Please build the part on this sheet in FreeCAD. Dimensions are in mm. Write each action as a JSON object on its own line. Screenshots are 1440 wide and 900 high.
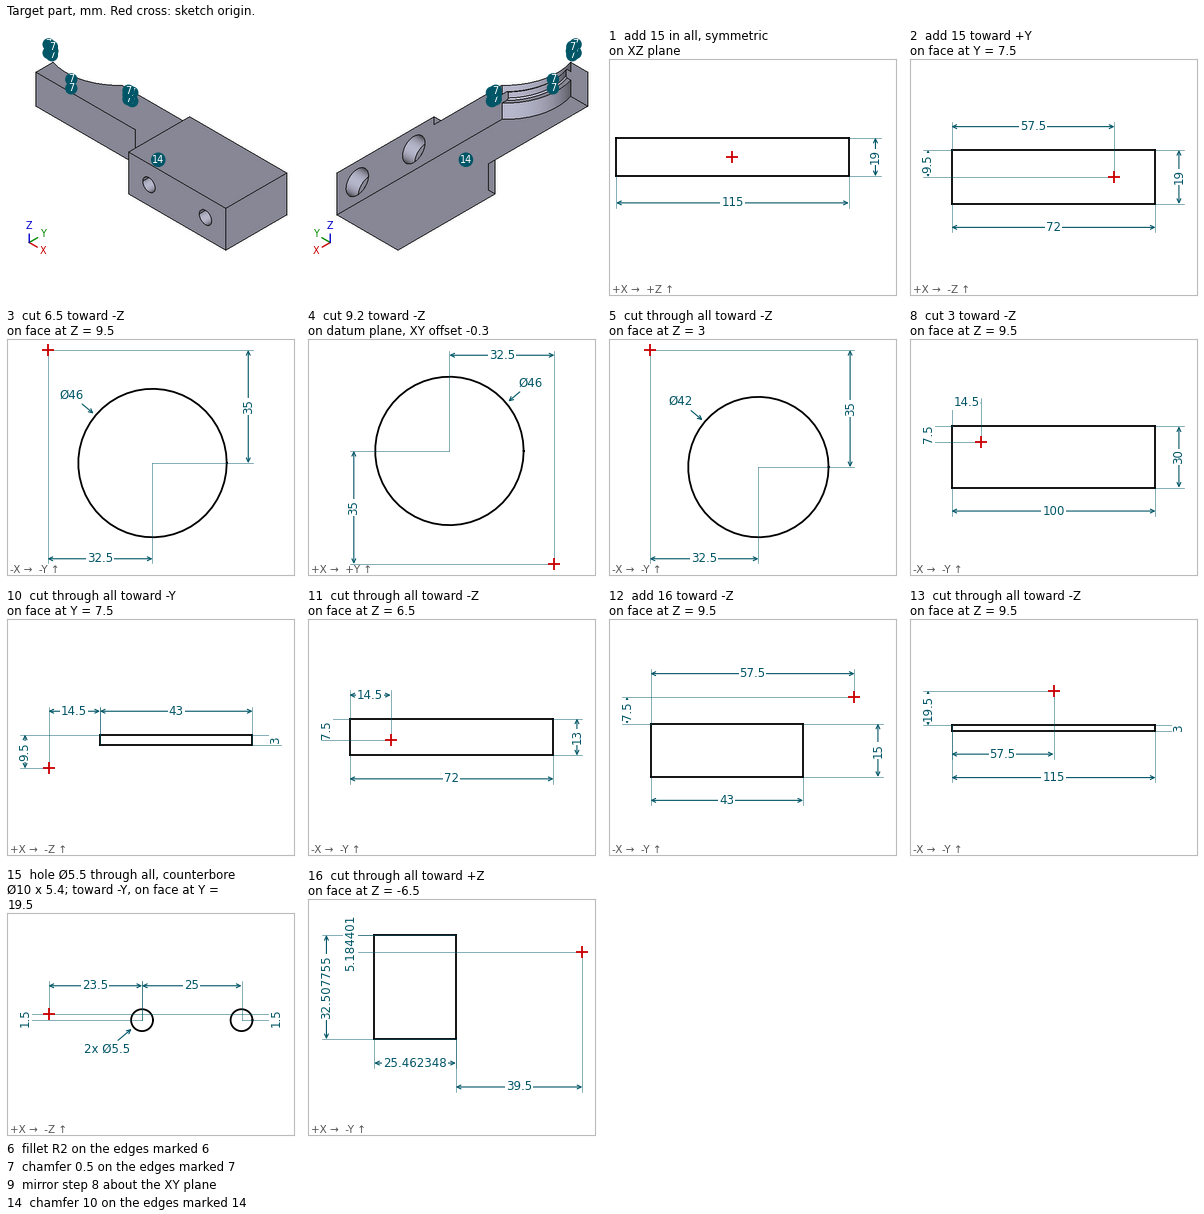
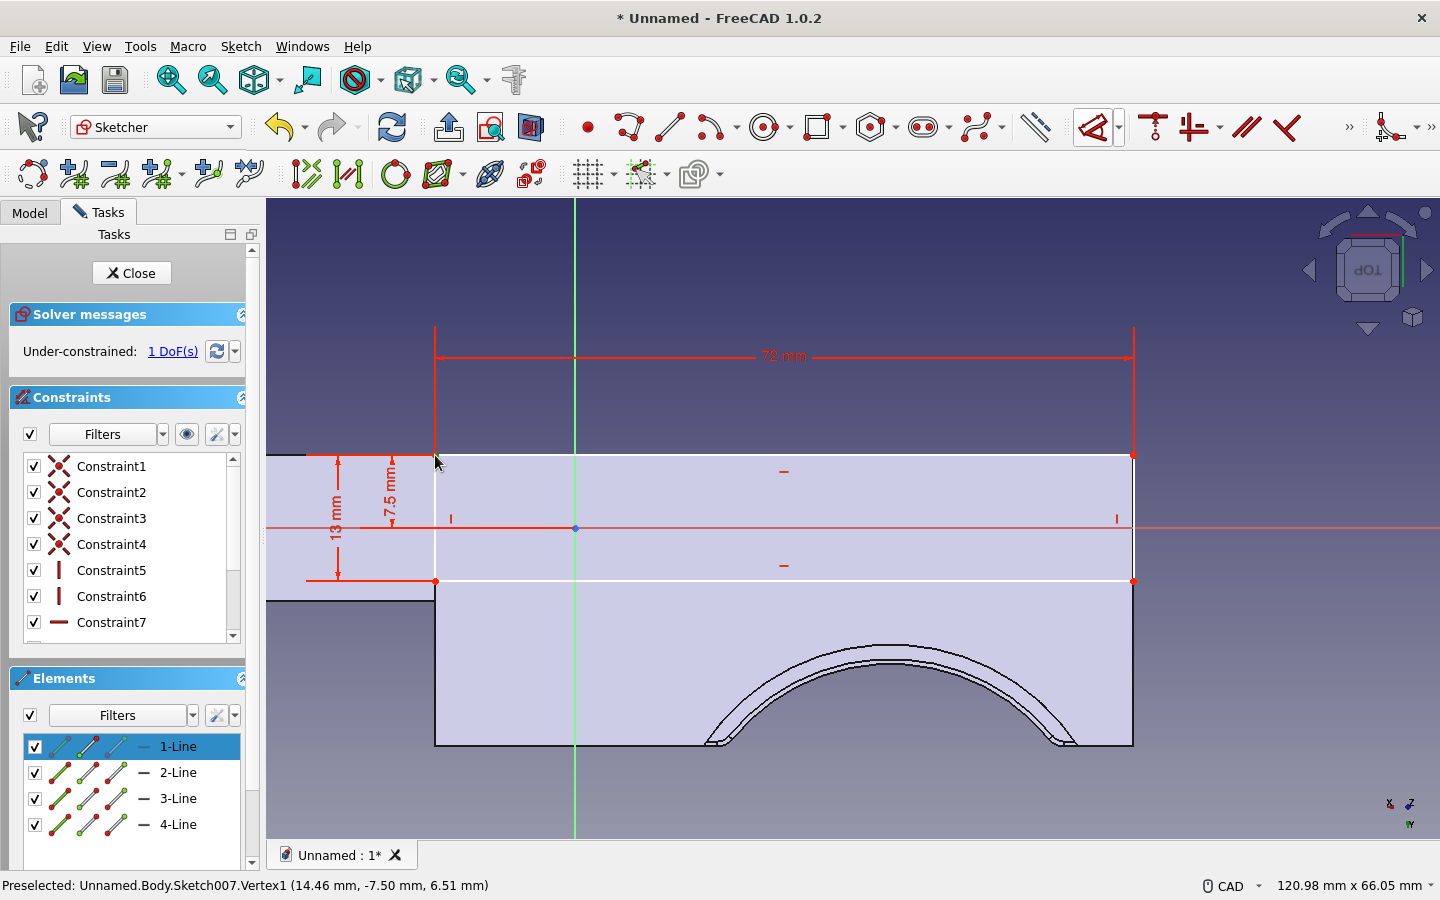
{"action": "left_click", "coordinate": [1118, 128]}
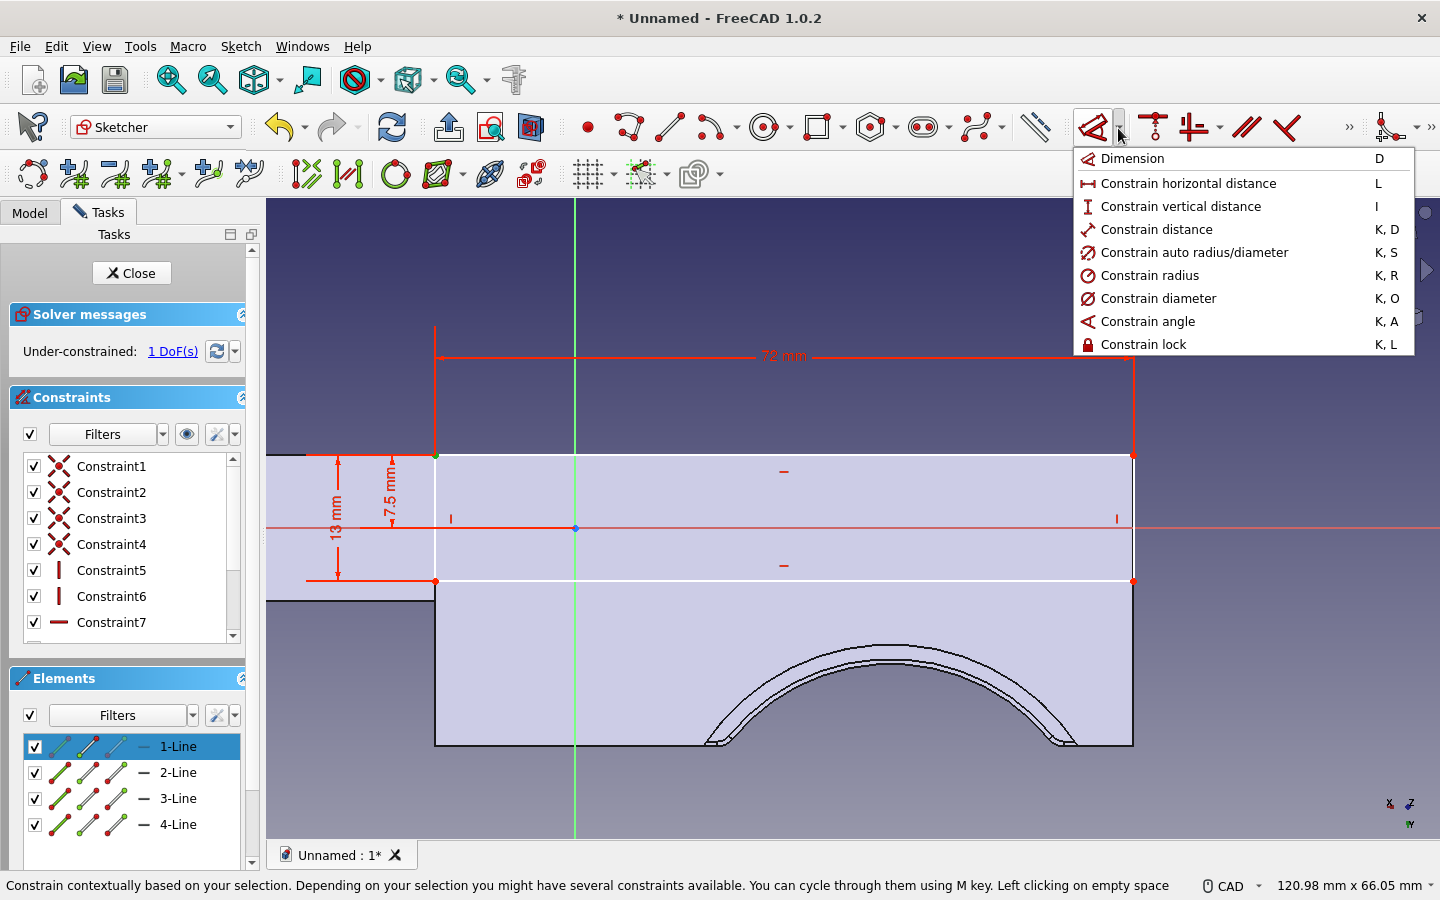
{"action": "left_click", "coordinate": [1244, 184]}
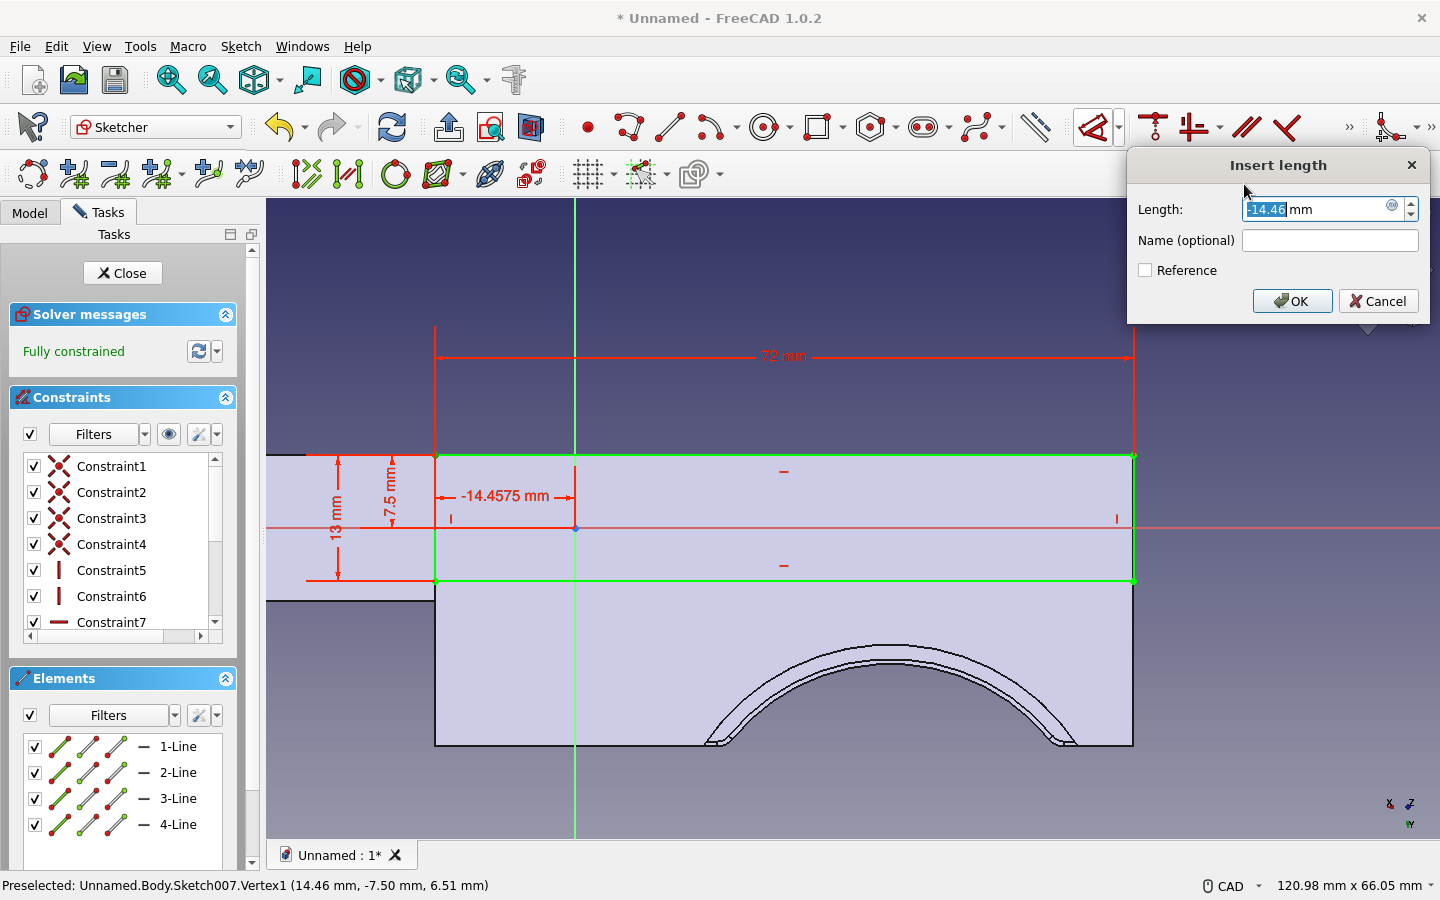
{"action": "type", "text": "-14.5"}
{"action": "key", "text": "Return"}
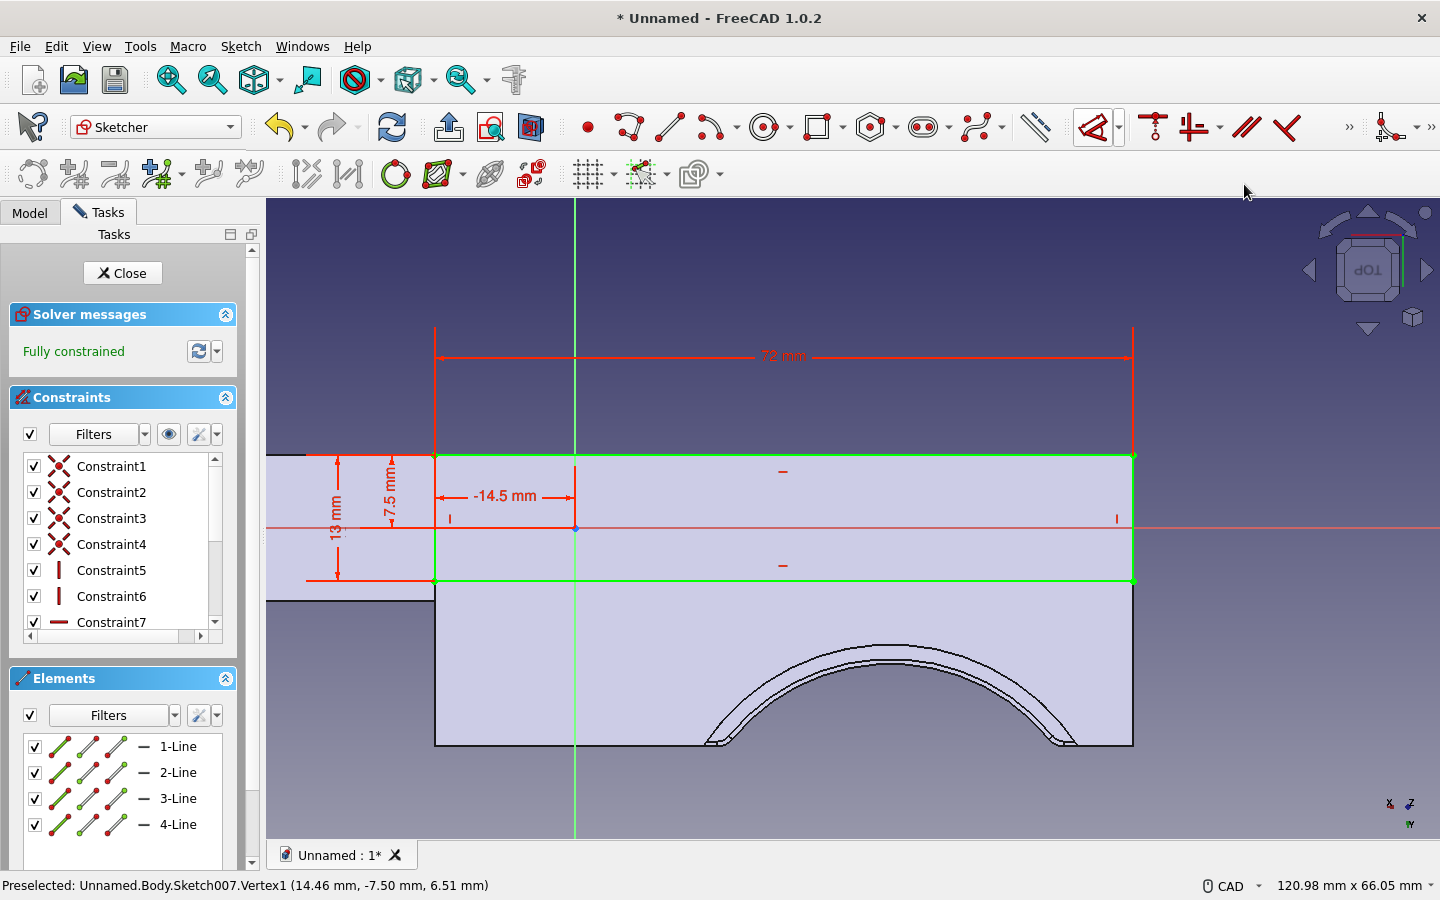
{"action": "left_click", "coordinate": [123, 273]}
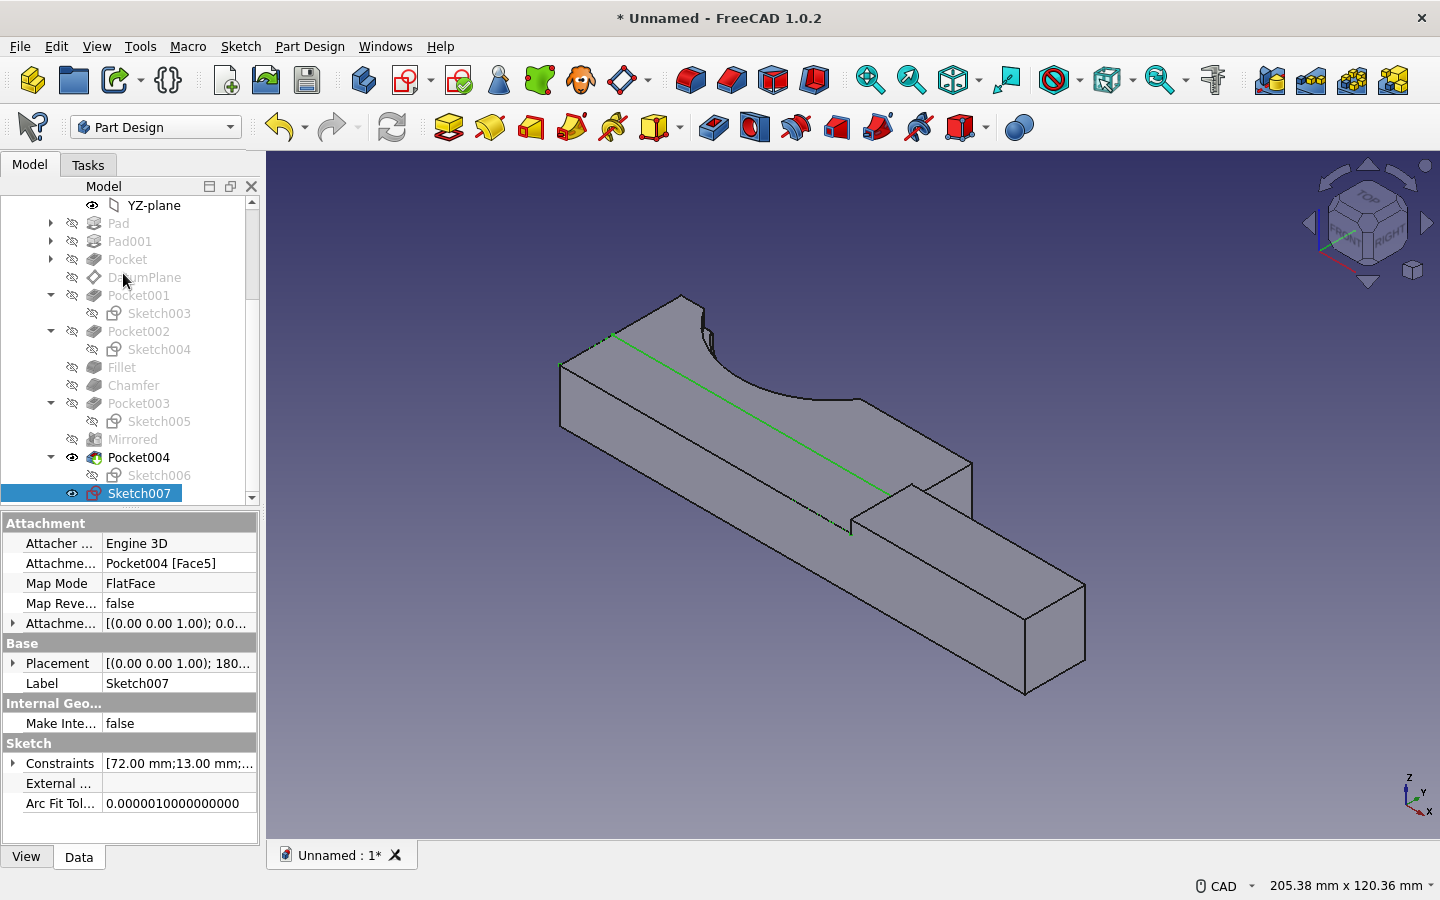
{"action": "left_click", "coordinate": [714, 128]}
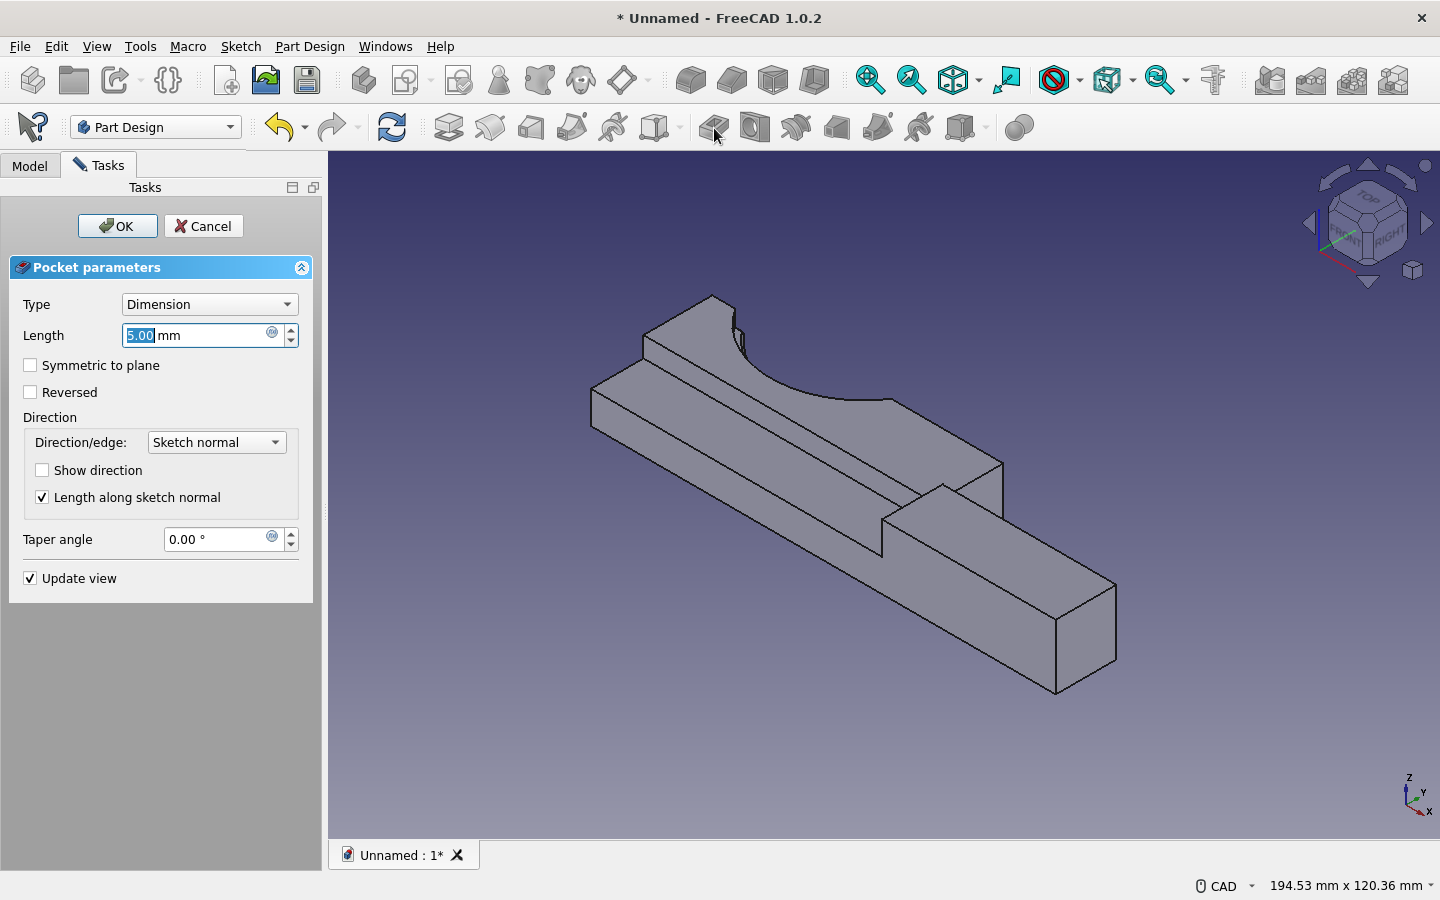
{"action": "left_click", "coordinate": [210, 304]}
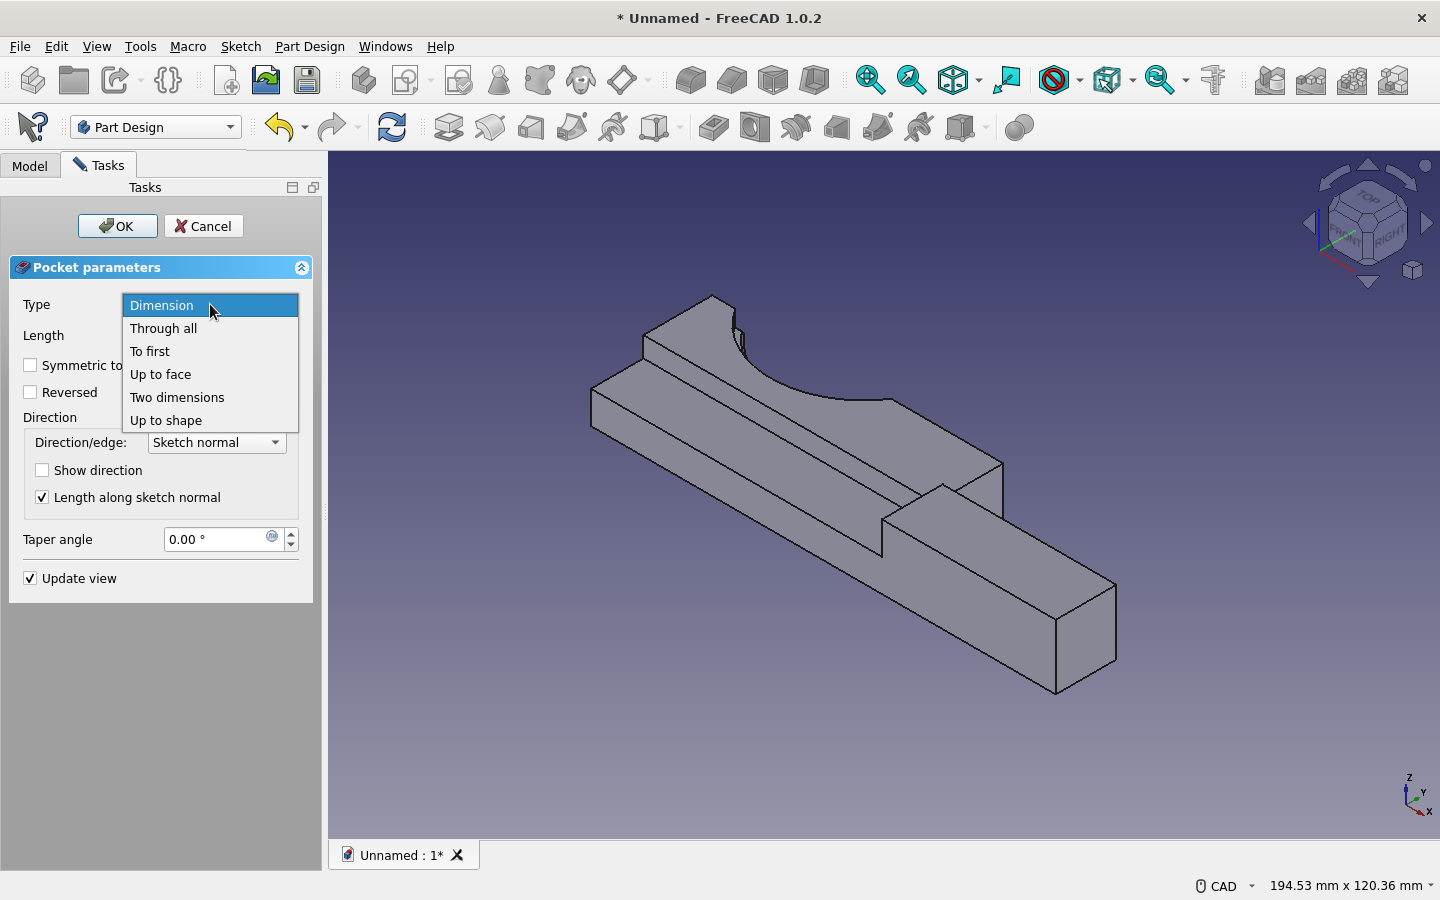
{"action": "left_click", "coordinate": [208, 328]}